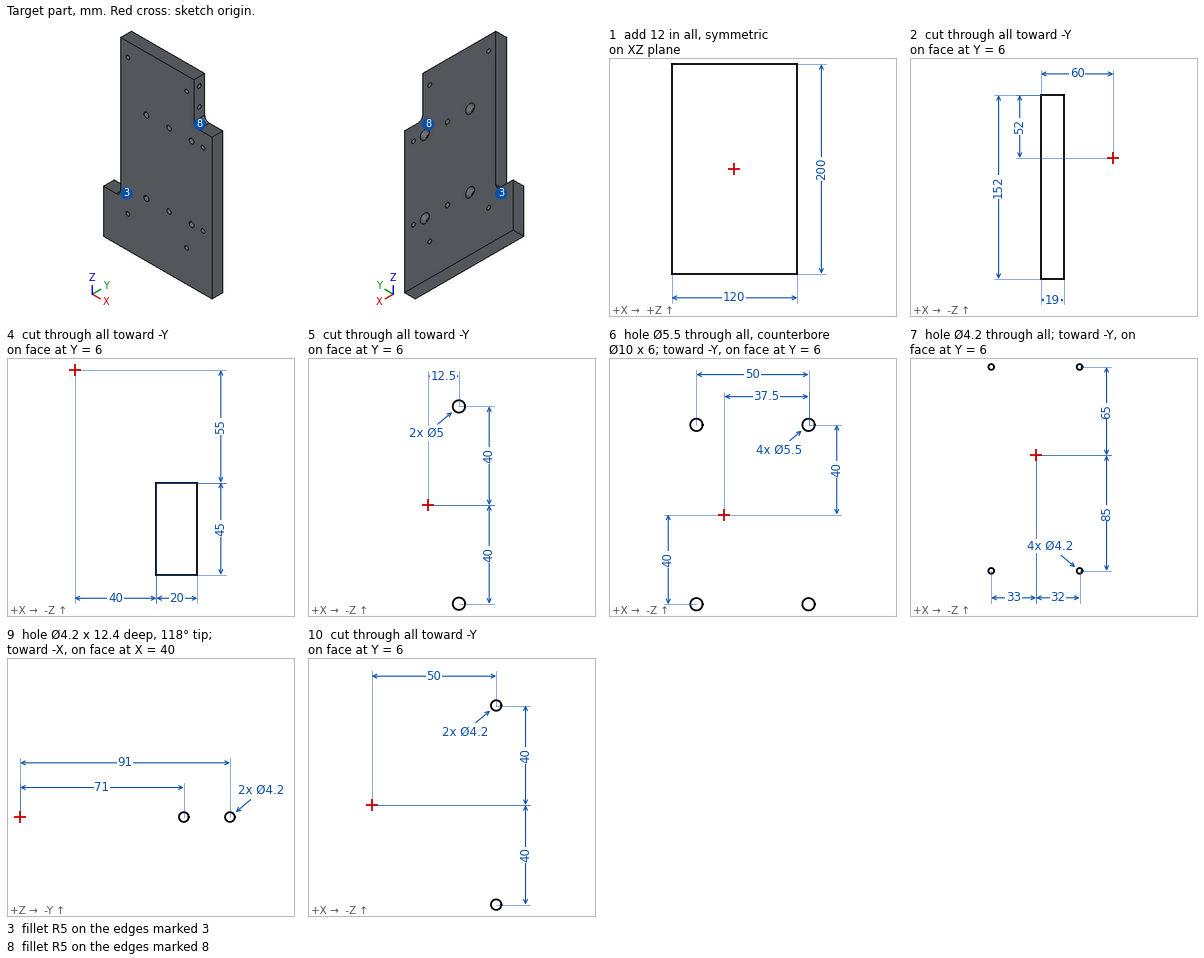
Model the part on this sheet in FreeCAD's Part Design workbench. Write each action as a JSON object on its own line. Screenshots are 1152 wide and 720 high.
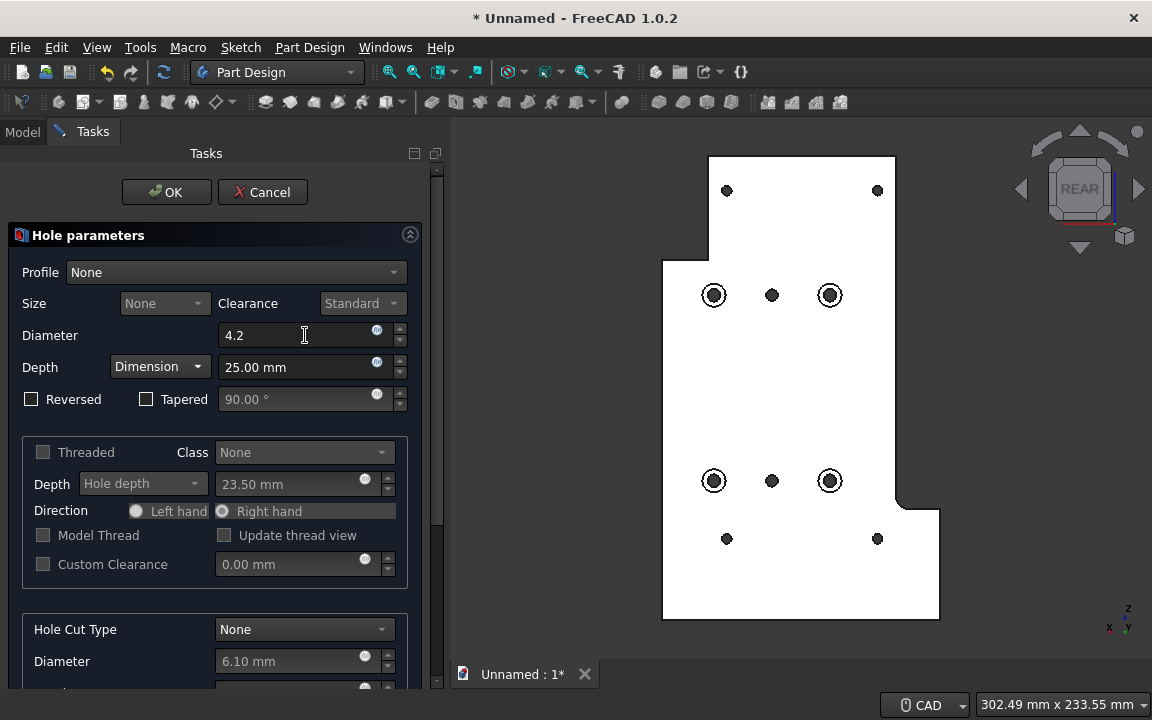
{"action": "left_click", "coordinate": [161, 366]}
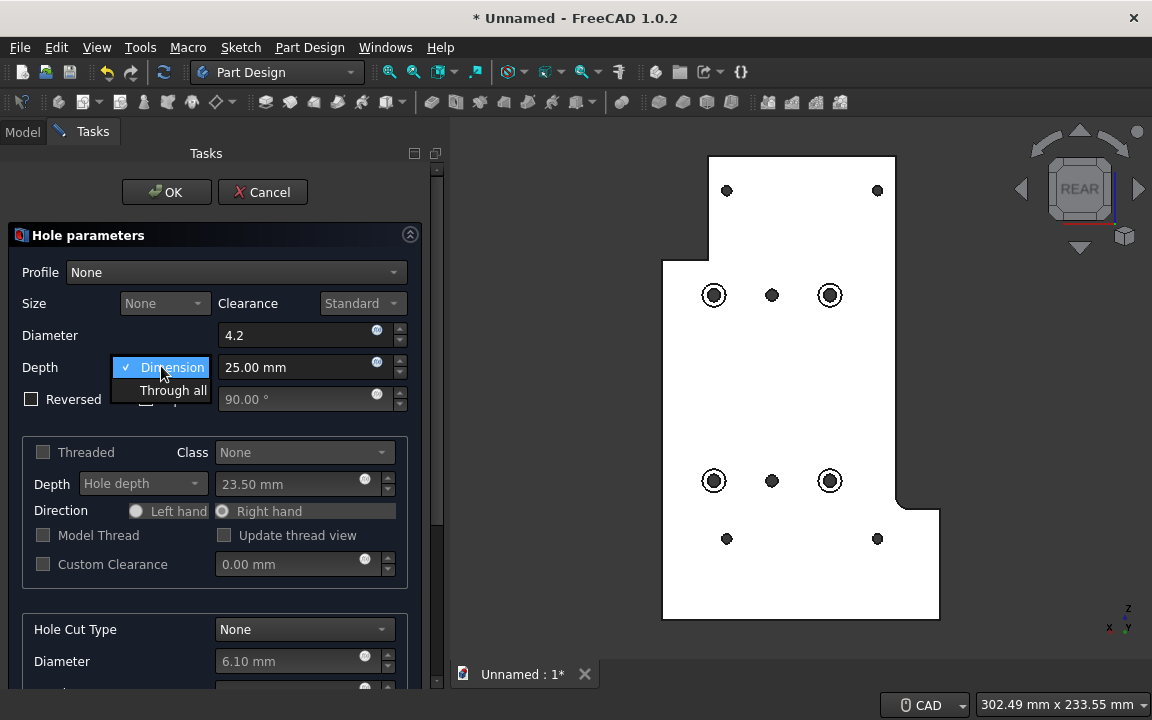
{"action": "left_click", "coordinate": [160, 390]}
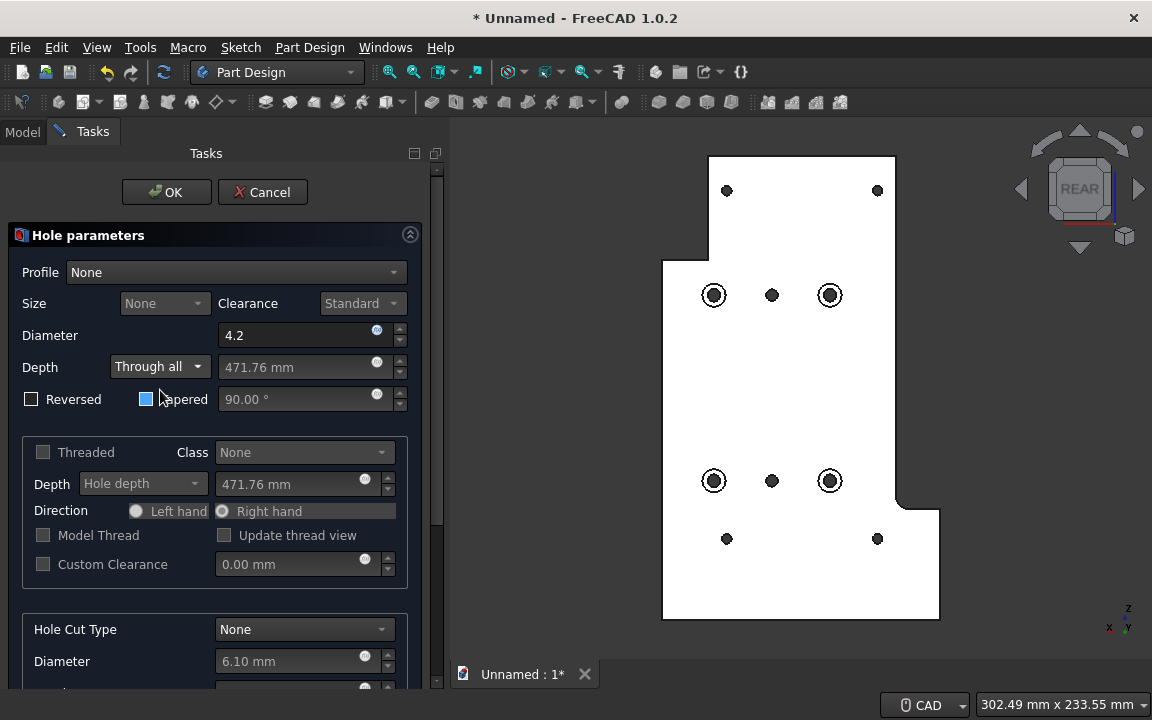
{"action": "left_click", "coordinate": [167, 192]}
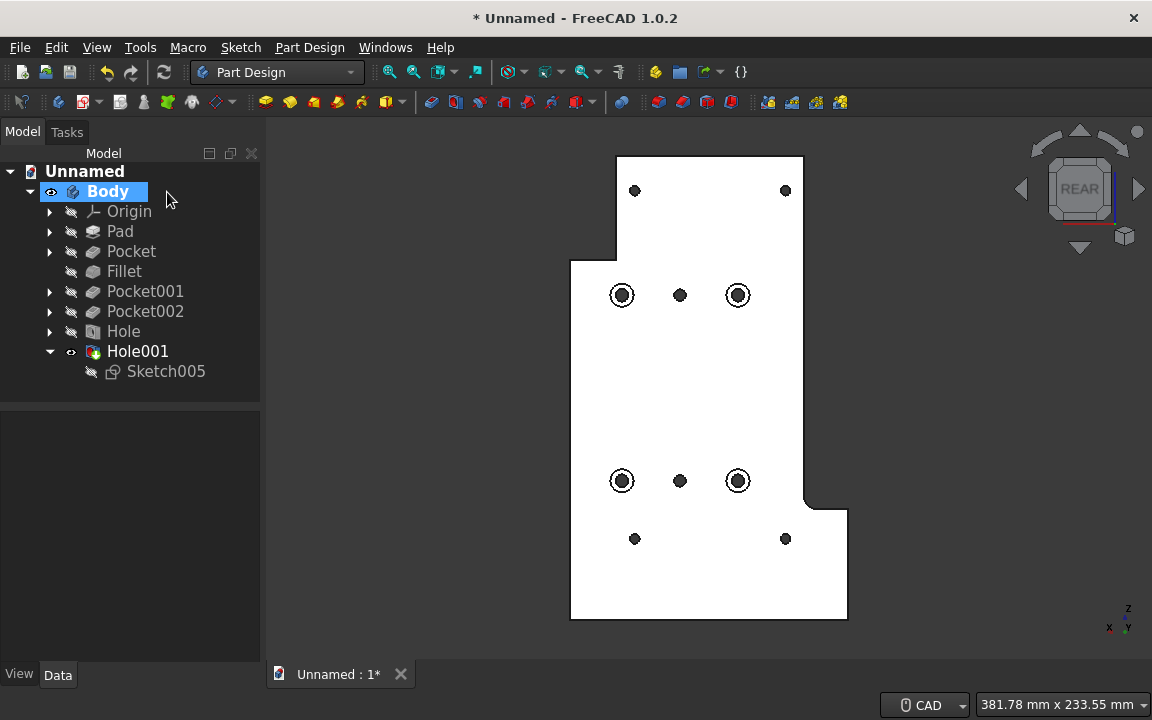
{"action": "key", "text": "0"}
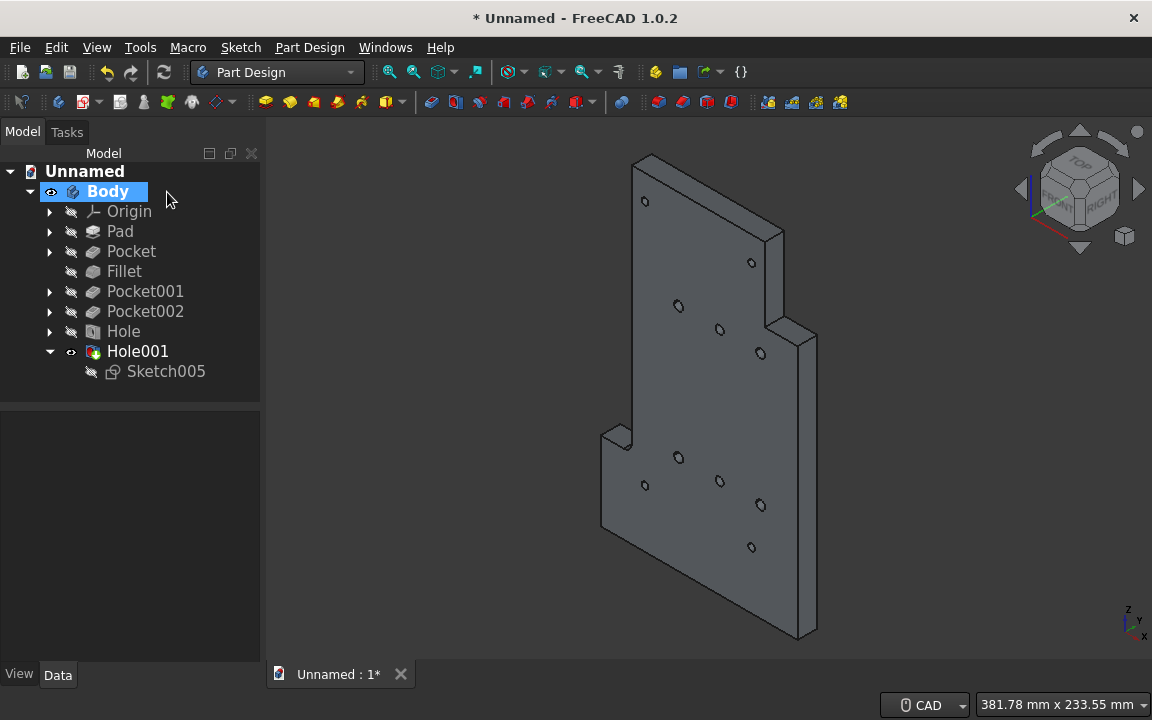
{"action": "key", "text": "2"}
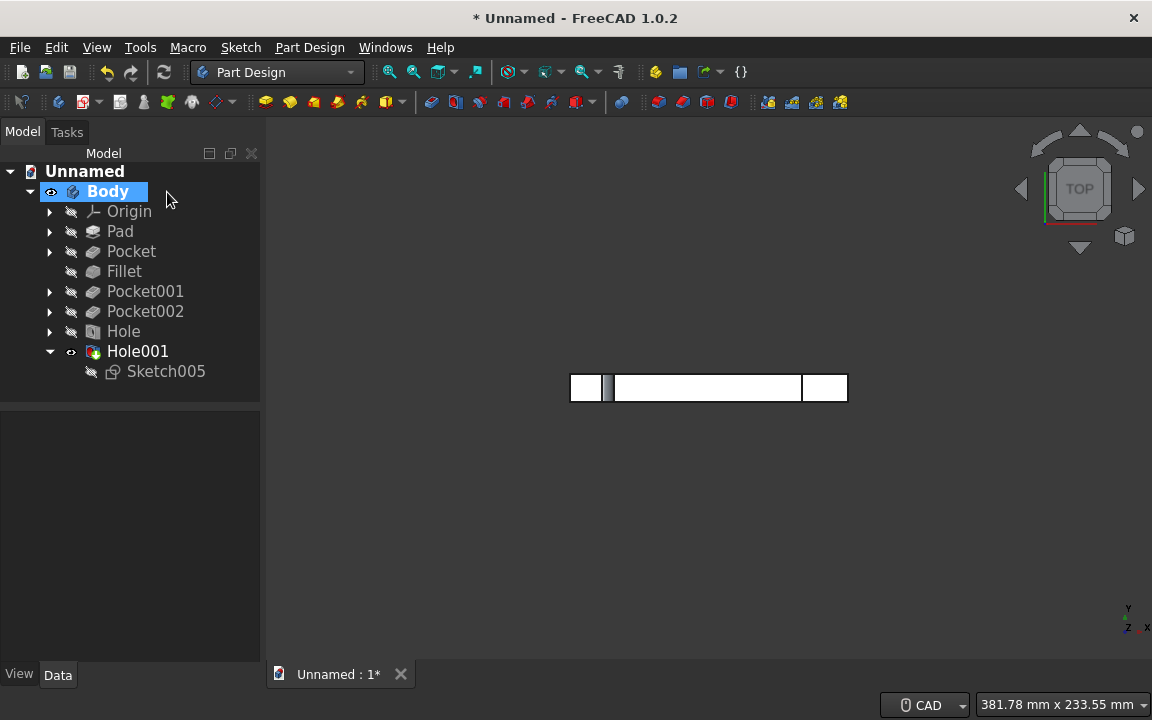
{"action": "left_click", "coordinate": [390, 72]}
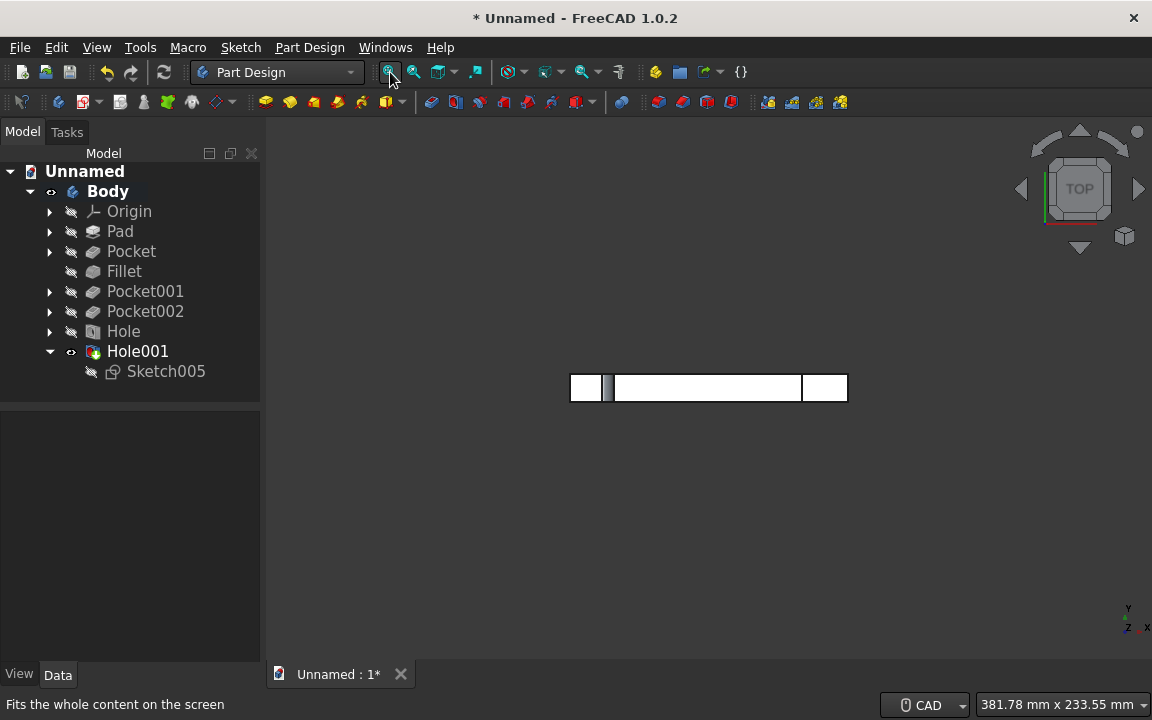
{"action": "key", "text": "1"}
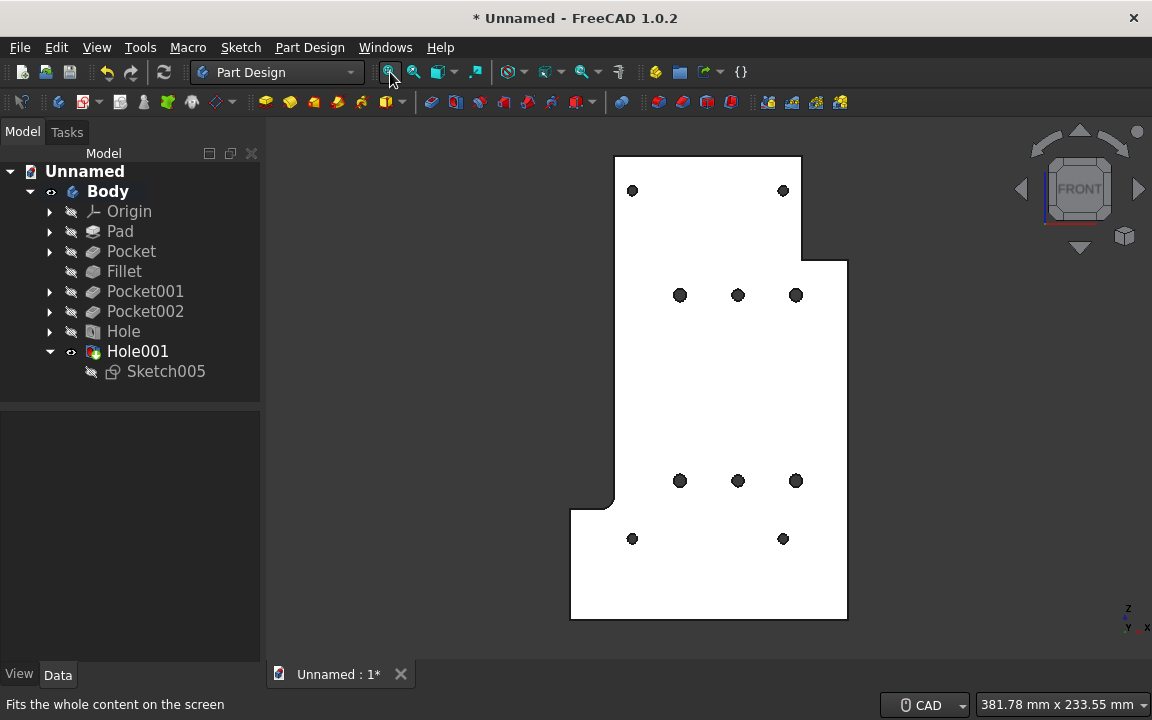
{"action": "key", "text": "3"}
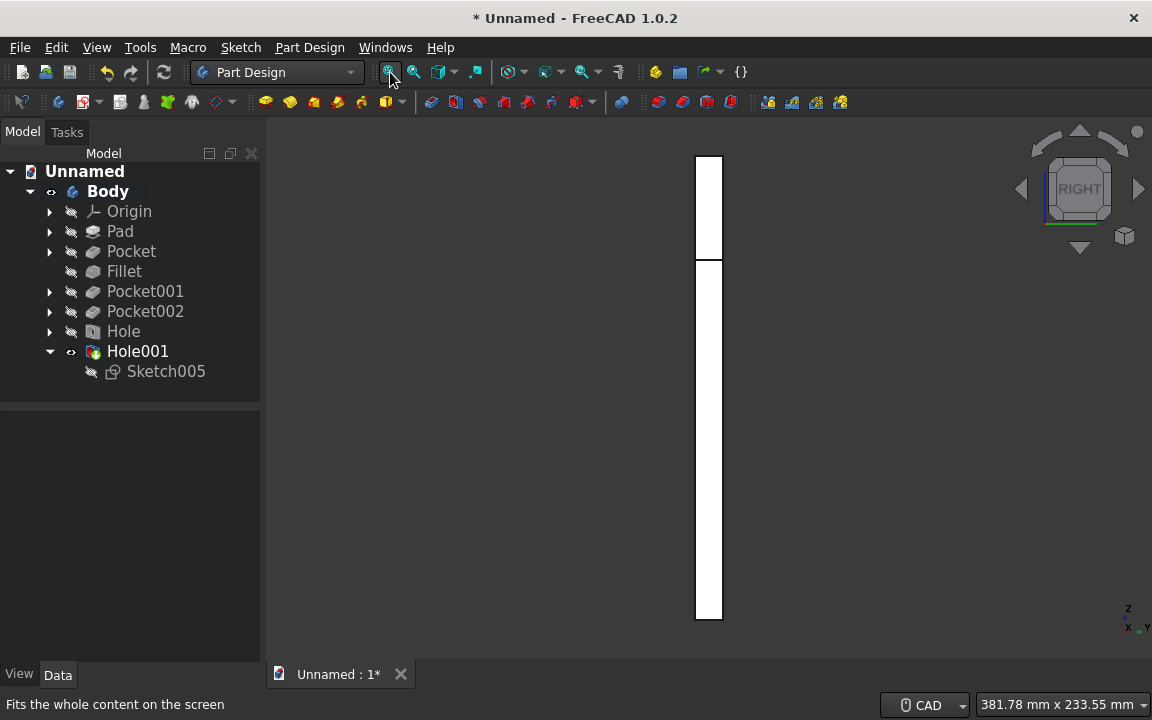
{"action": "key", "text": "5"}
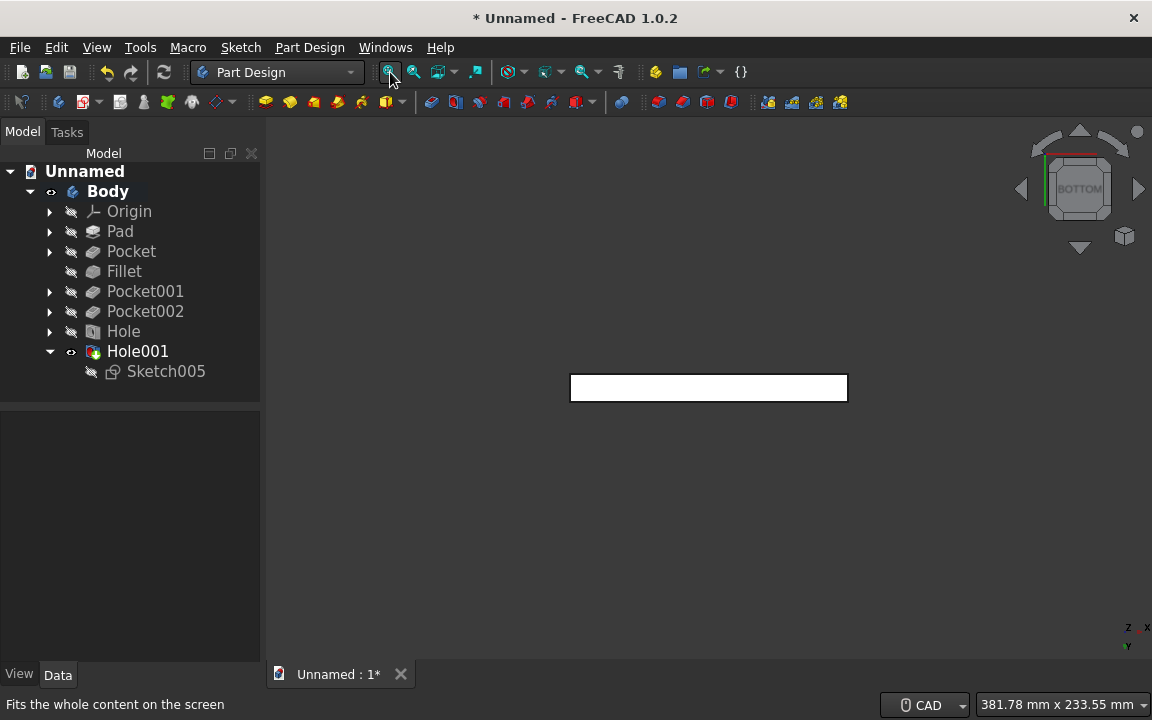
{"action": "left_click", "coordinate": [390, 72]}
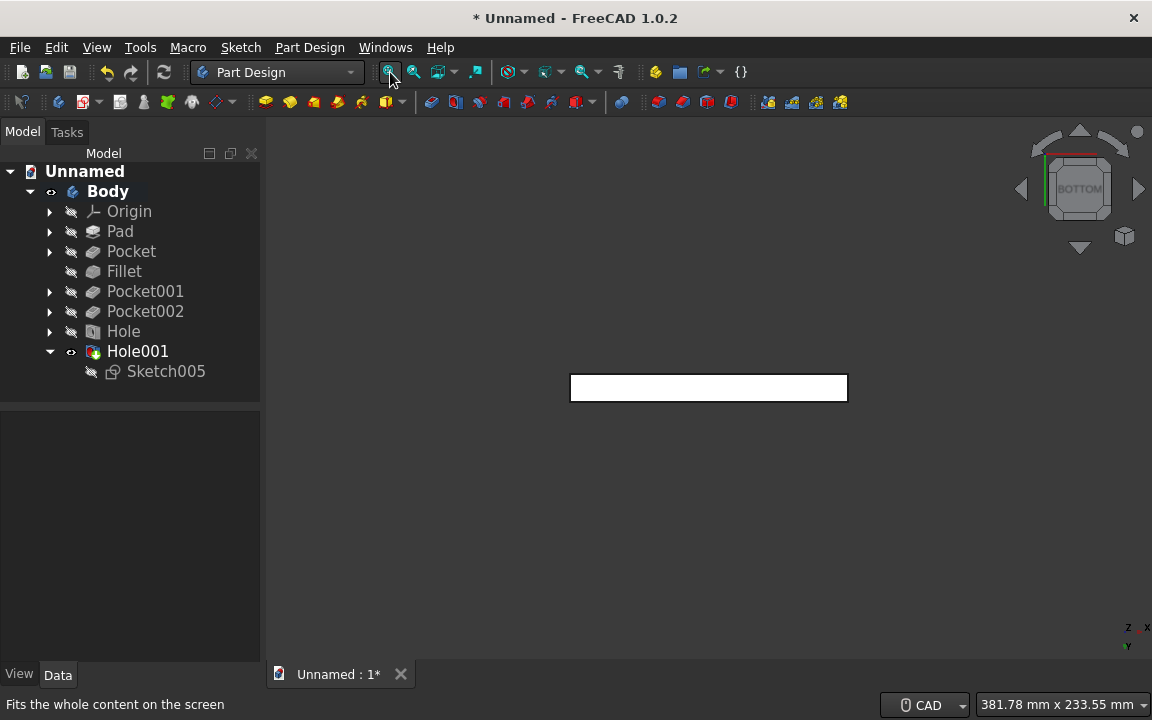
{"action": "key", "text": "4"}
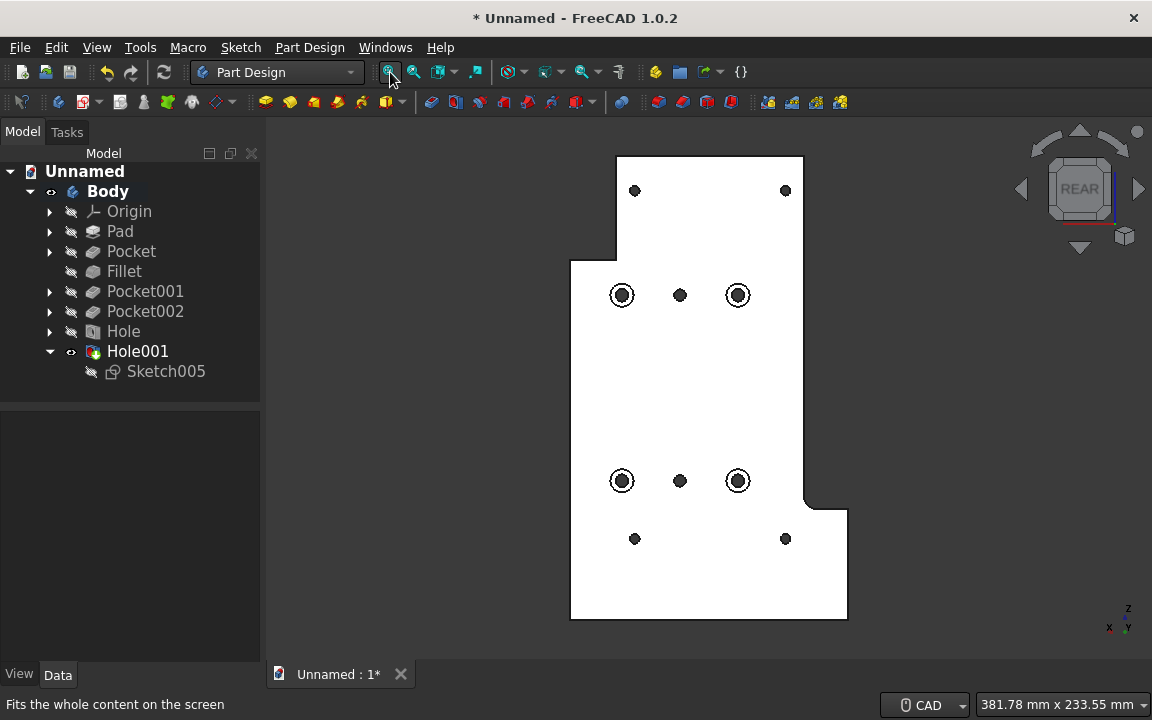
{"action": "key", "text": "6"}